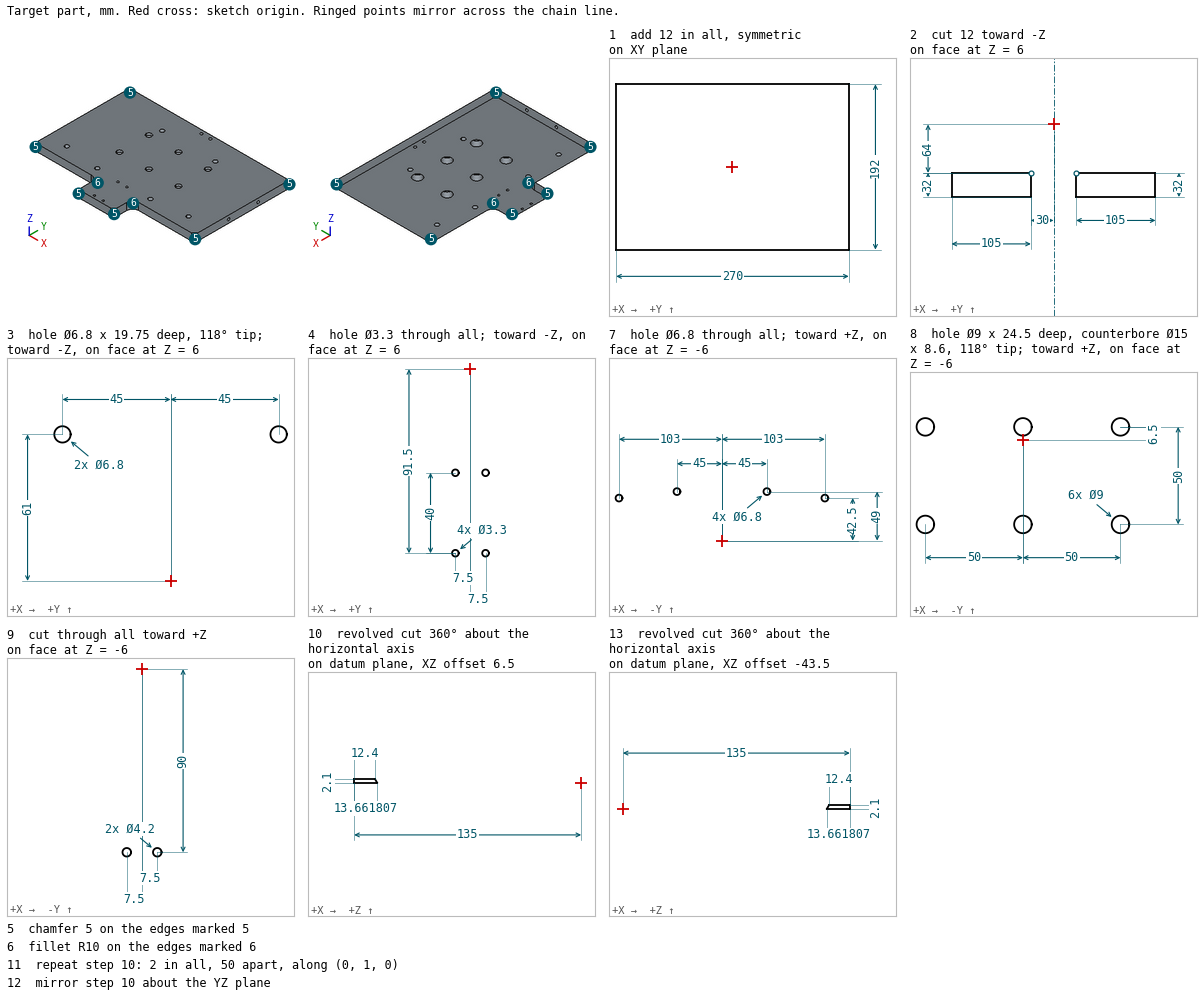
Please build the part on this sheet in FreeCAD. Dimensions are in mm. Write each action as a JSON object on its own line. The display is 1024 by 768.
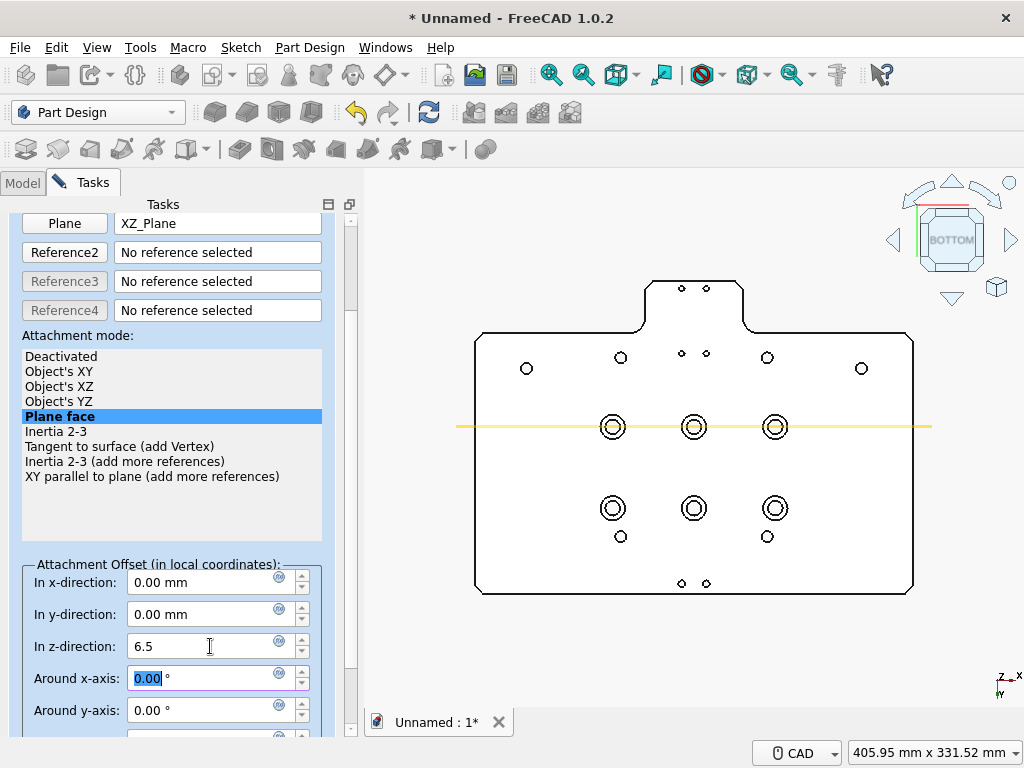
{"action": "scroll", "coordinate": [351, 475], "scroll_direction": "up", "scroll_amount": 3}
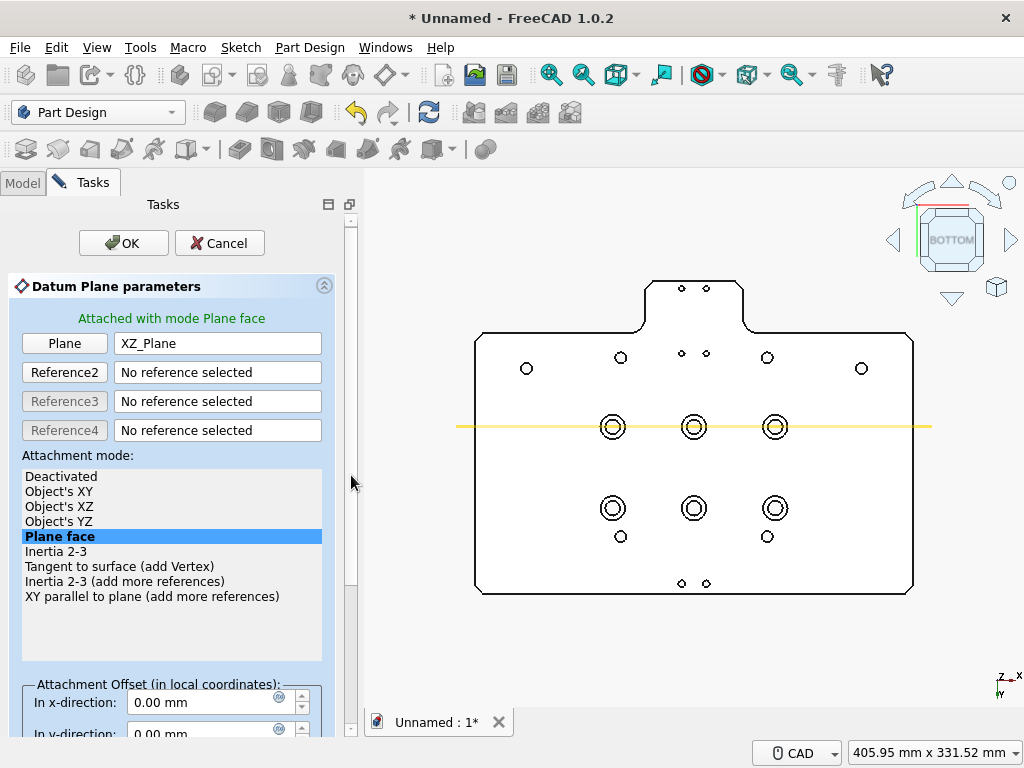
{"action": "left_click", "coordinate": [124, 243]}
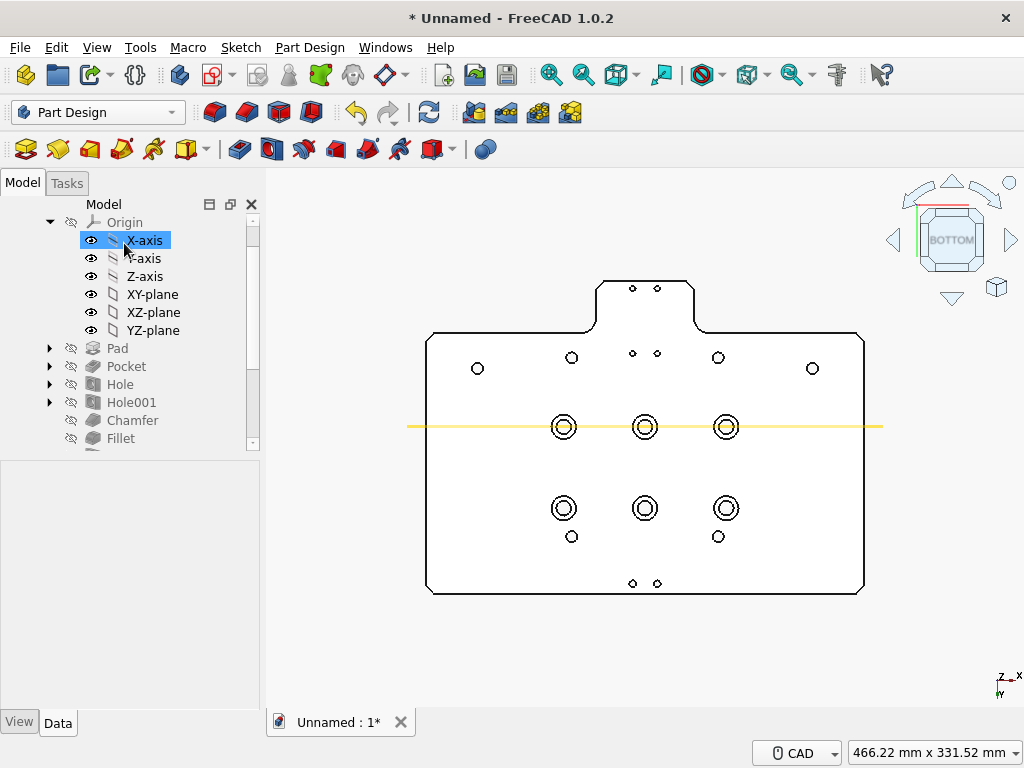
{"action": "scroll", "coordinate": [140, 326], "scroll_direction": "down", "scroll_amount": 3}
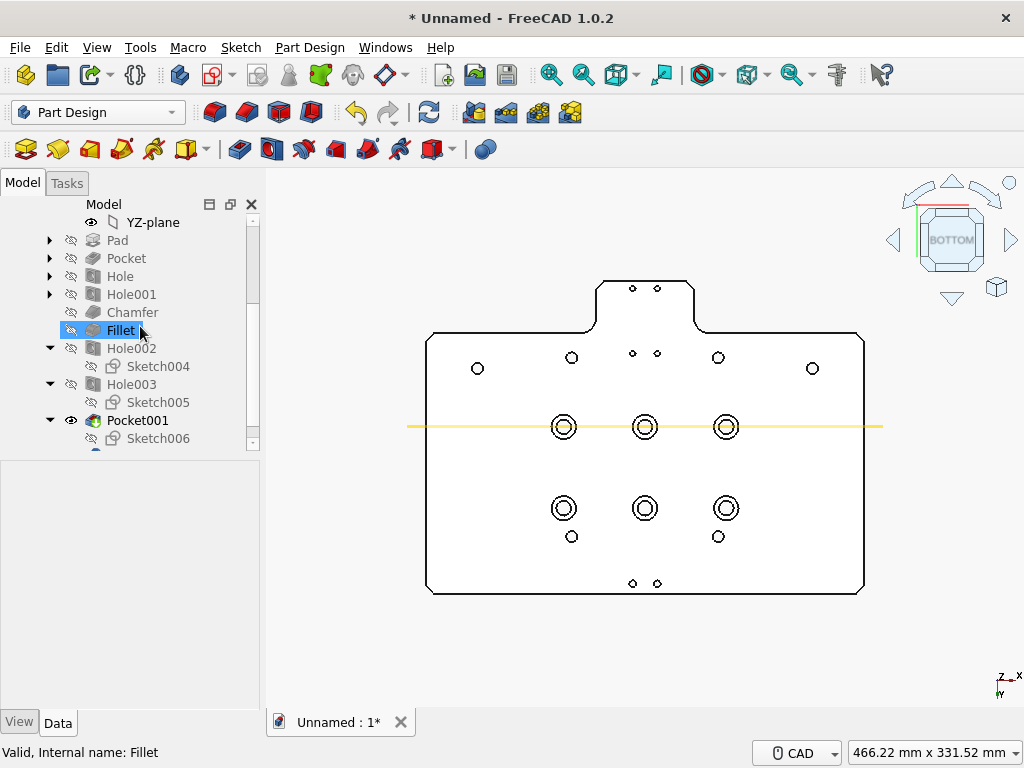
{"action": "left_click", "coordinate": [116, 438]}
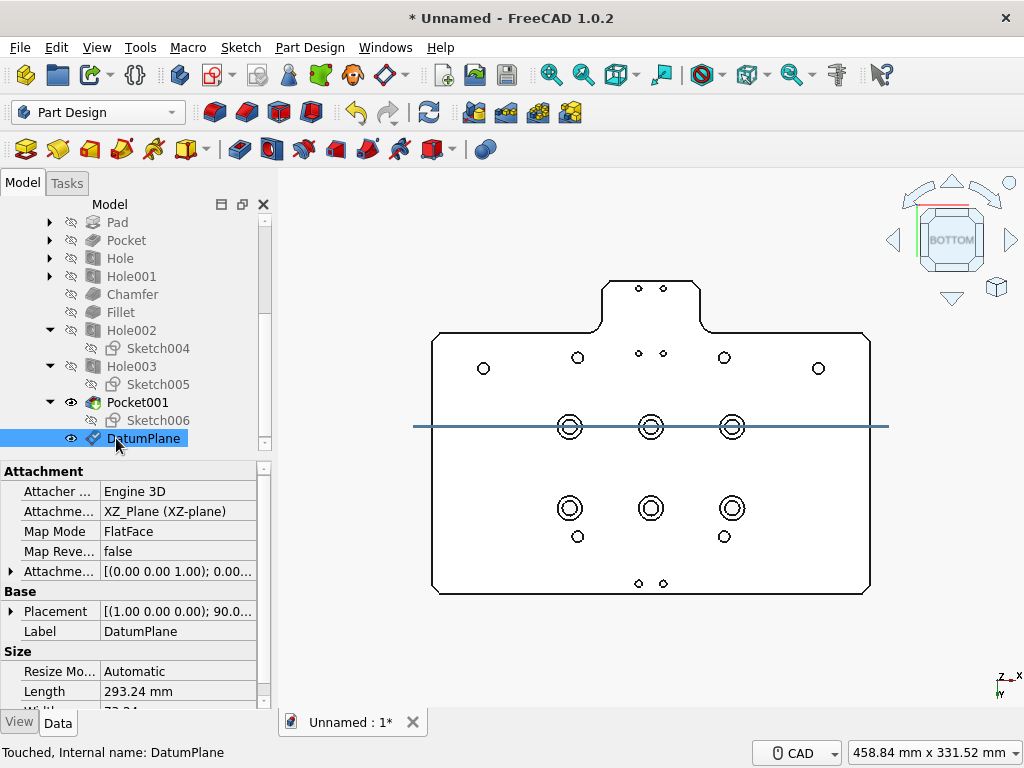
{"action": "left_click", "coordinate": [212, 76]}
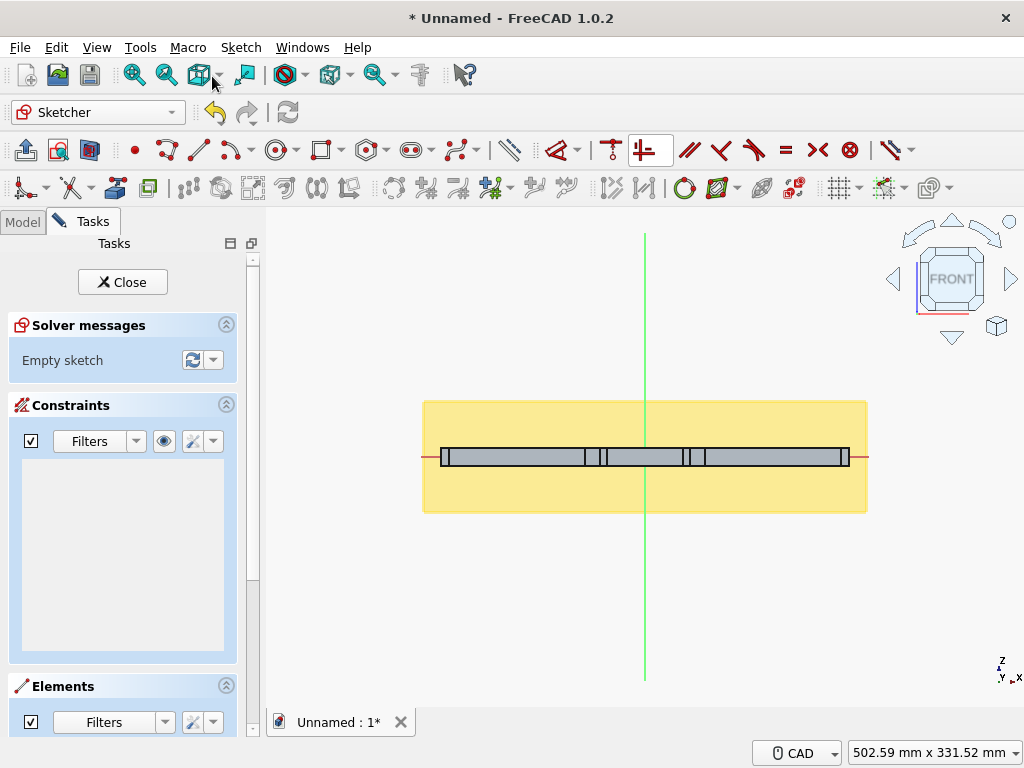
{"action": "left_click", "coordinate": [90, 150]}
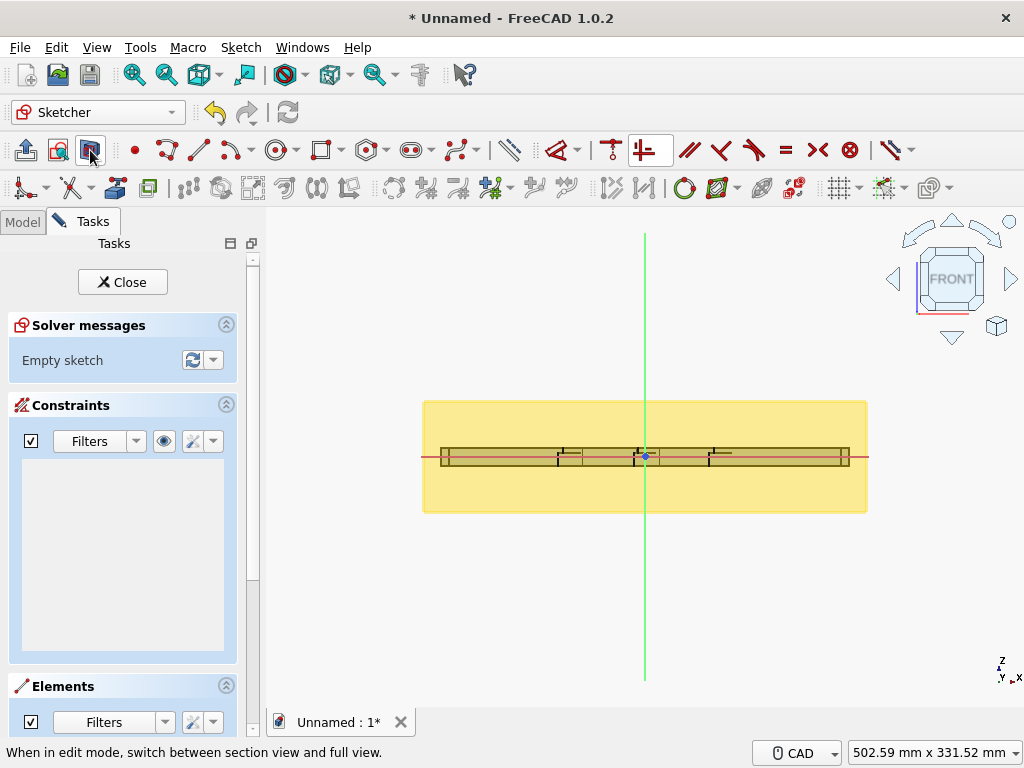
{"action": "scroll", "coordinate": [445, 455], "scroll_direction": "up", "scroll_amount": 15}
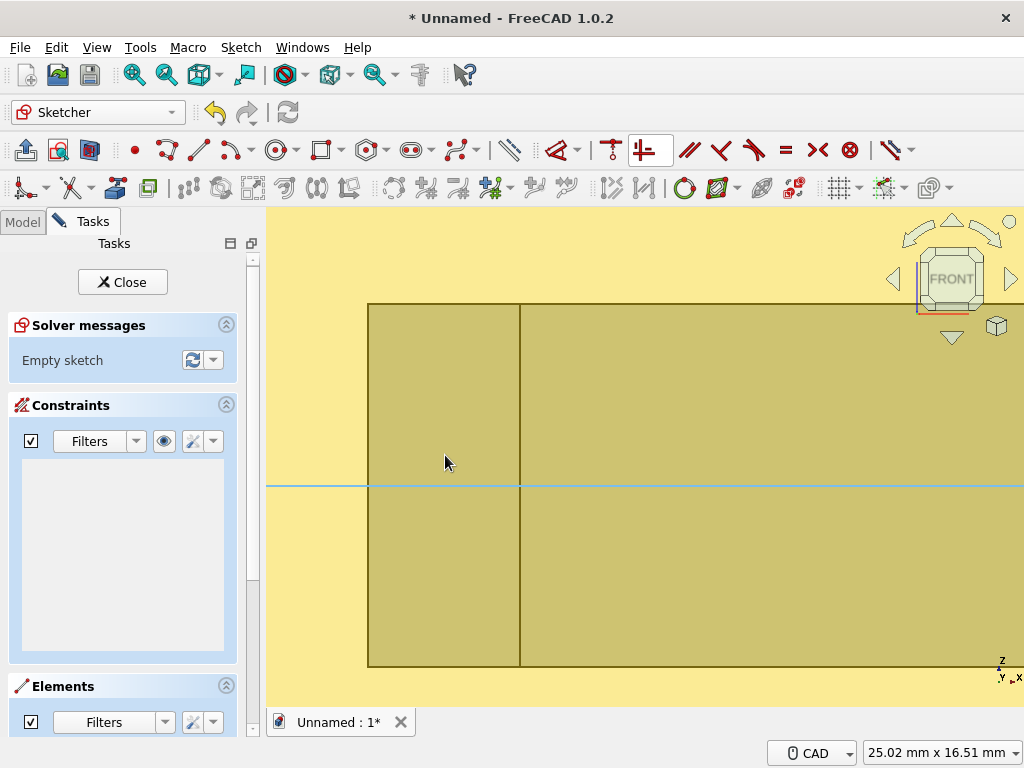
{"action": "key", "text": "g m"}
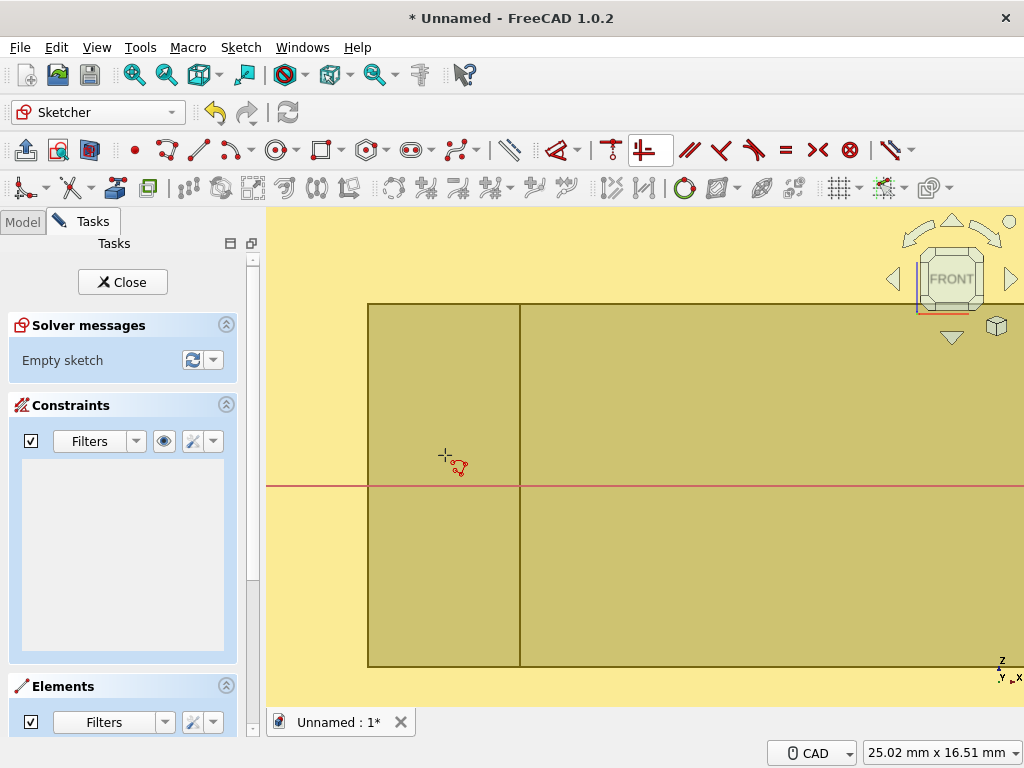
{"action": "left_click", "coordinate": [782, 486]}
{"action": "left_click", "coordinate": [368, 477]}
{"action": "left_click", "coordinate": [368, 422]}
{"action": "left_click", "coordinate": [744, 422]}
{"action": "left_click", "coordinate": [782, 486]}
{"action": "key", "text": "Escape"}
{"action": "key", "text": "Escape"}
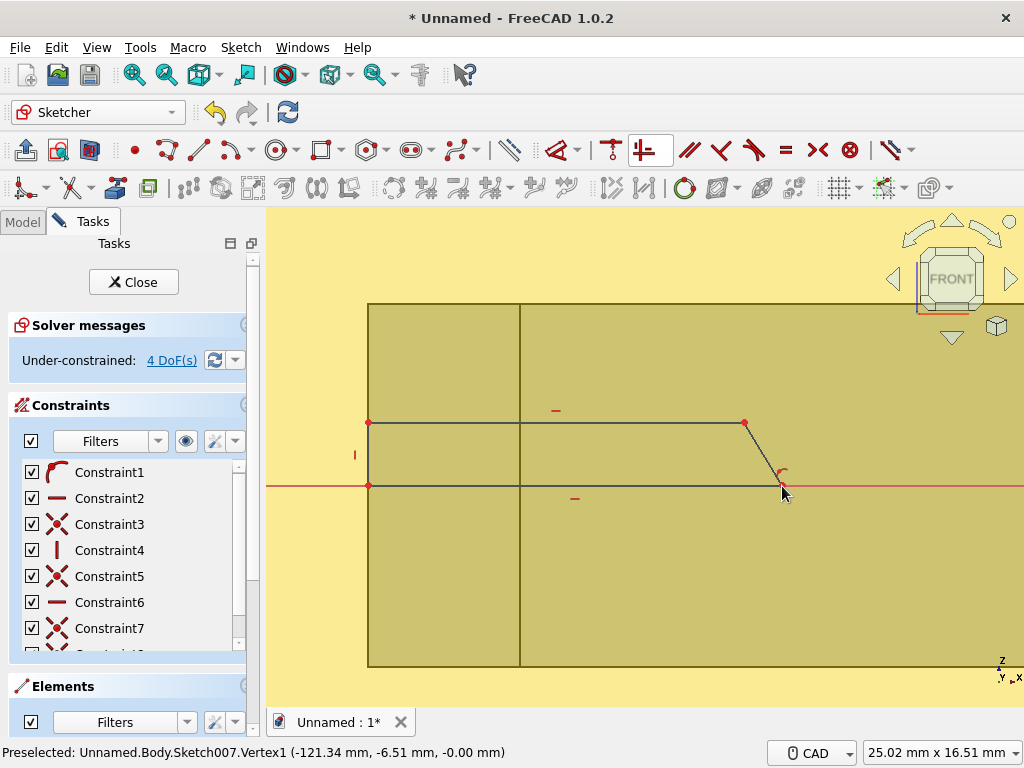
{"action": "key", "text": "d"}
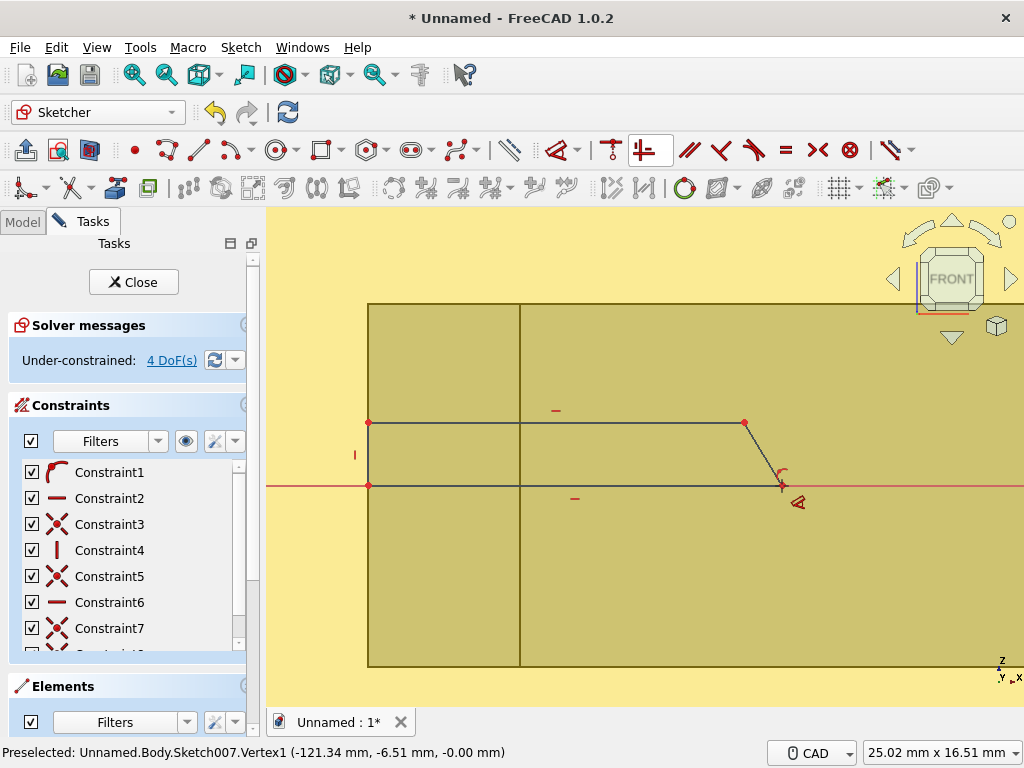
{"action": "left_click", "coordinate": [368, 467]}
{"action": "left_click", "coordinate": [334, 454]}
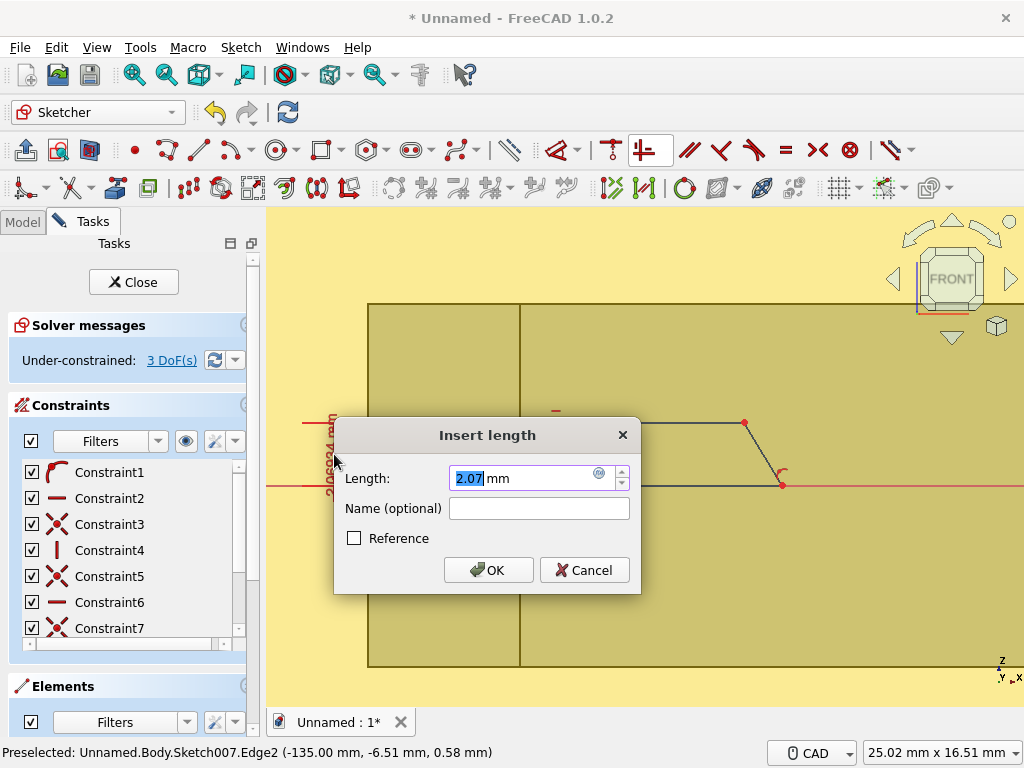
{"action": "type", "text": "2.1"}
{"action": "key", "text": "Return"}